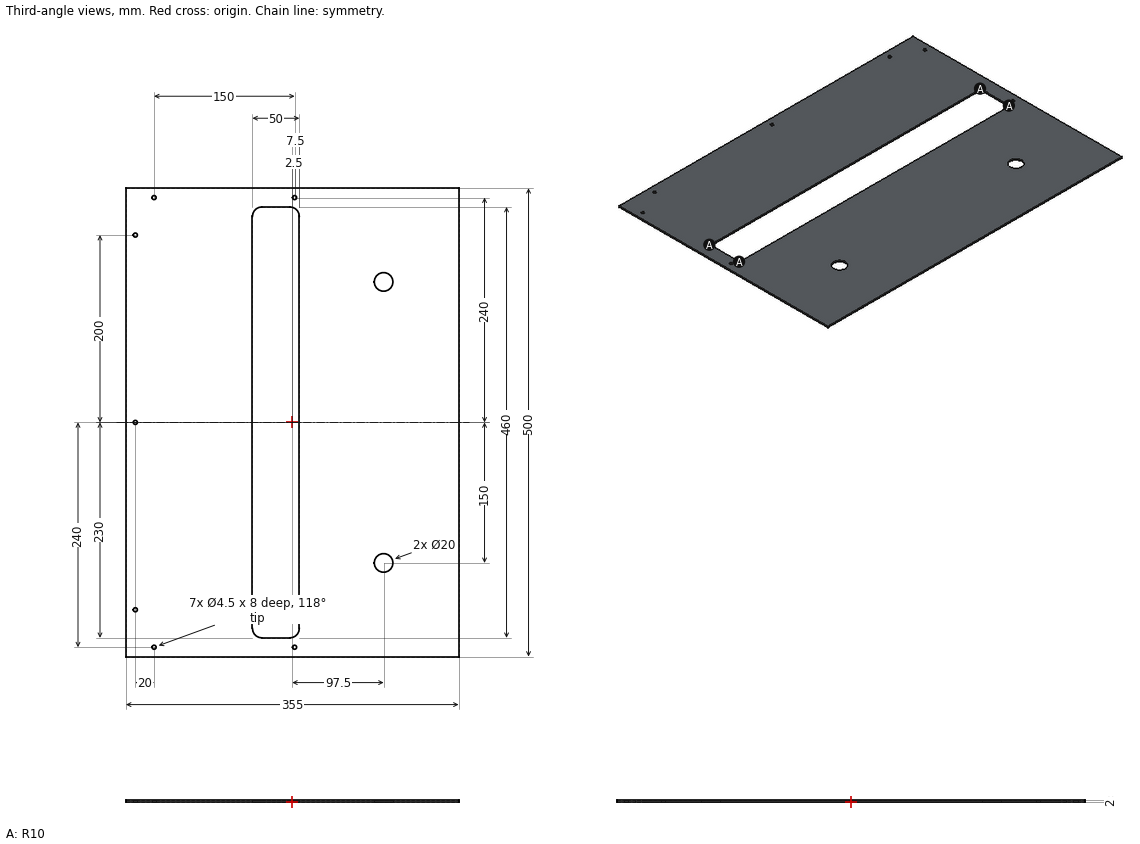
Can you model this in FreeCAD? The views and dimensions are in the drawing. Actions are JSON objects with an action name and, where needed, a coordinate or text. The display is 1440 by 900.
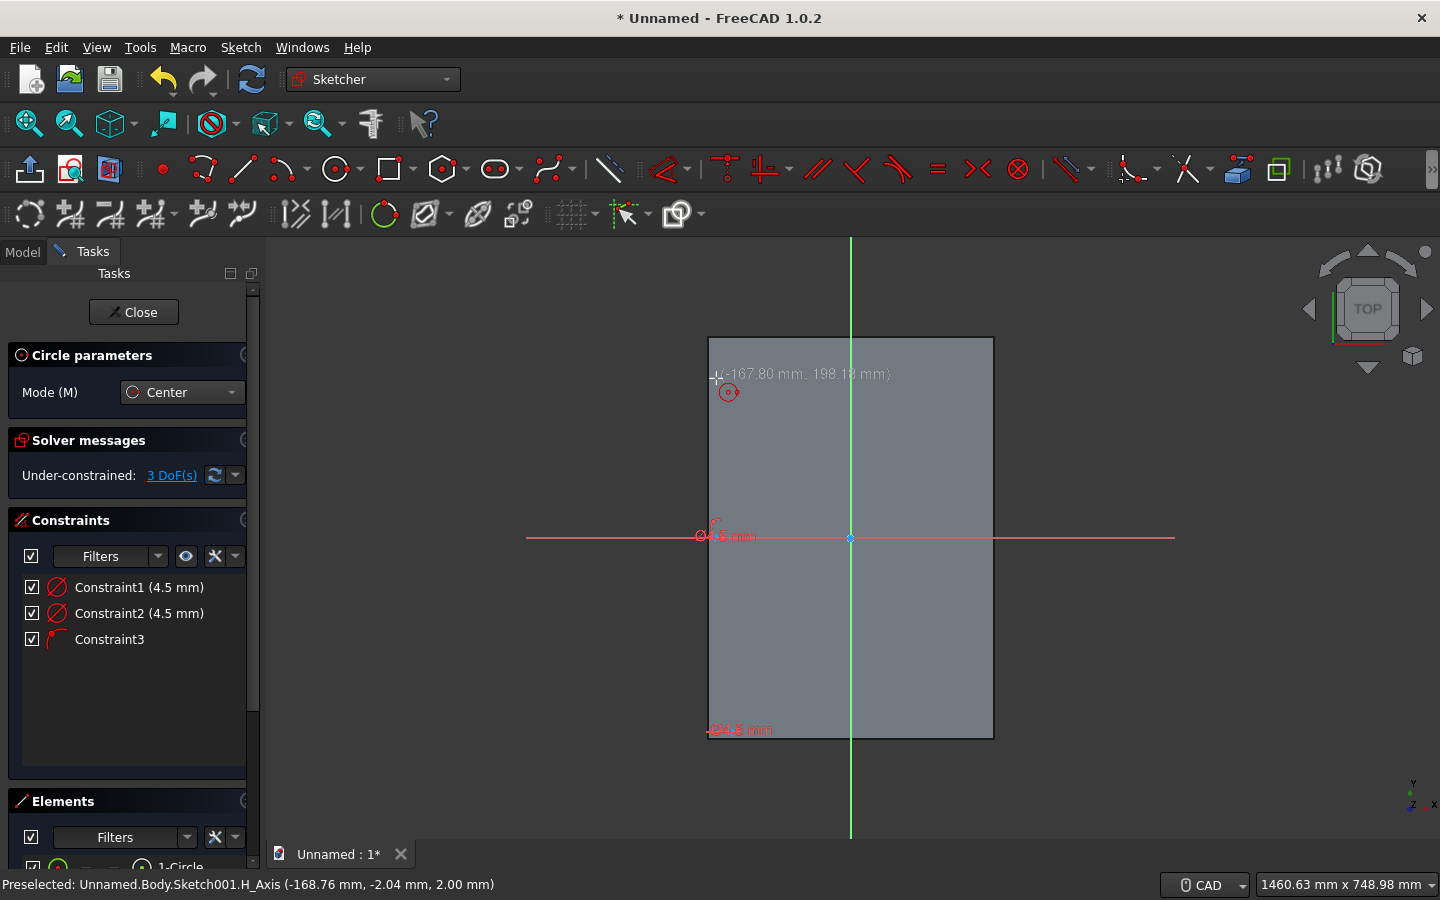
{"action": "left_click", "coordinate": [716, 378]}
{"action": "mouse_move", "coordinate": [718, 376]}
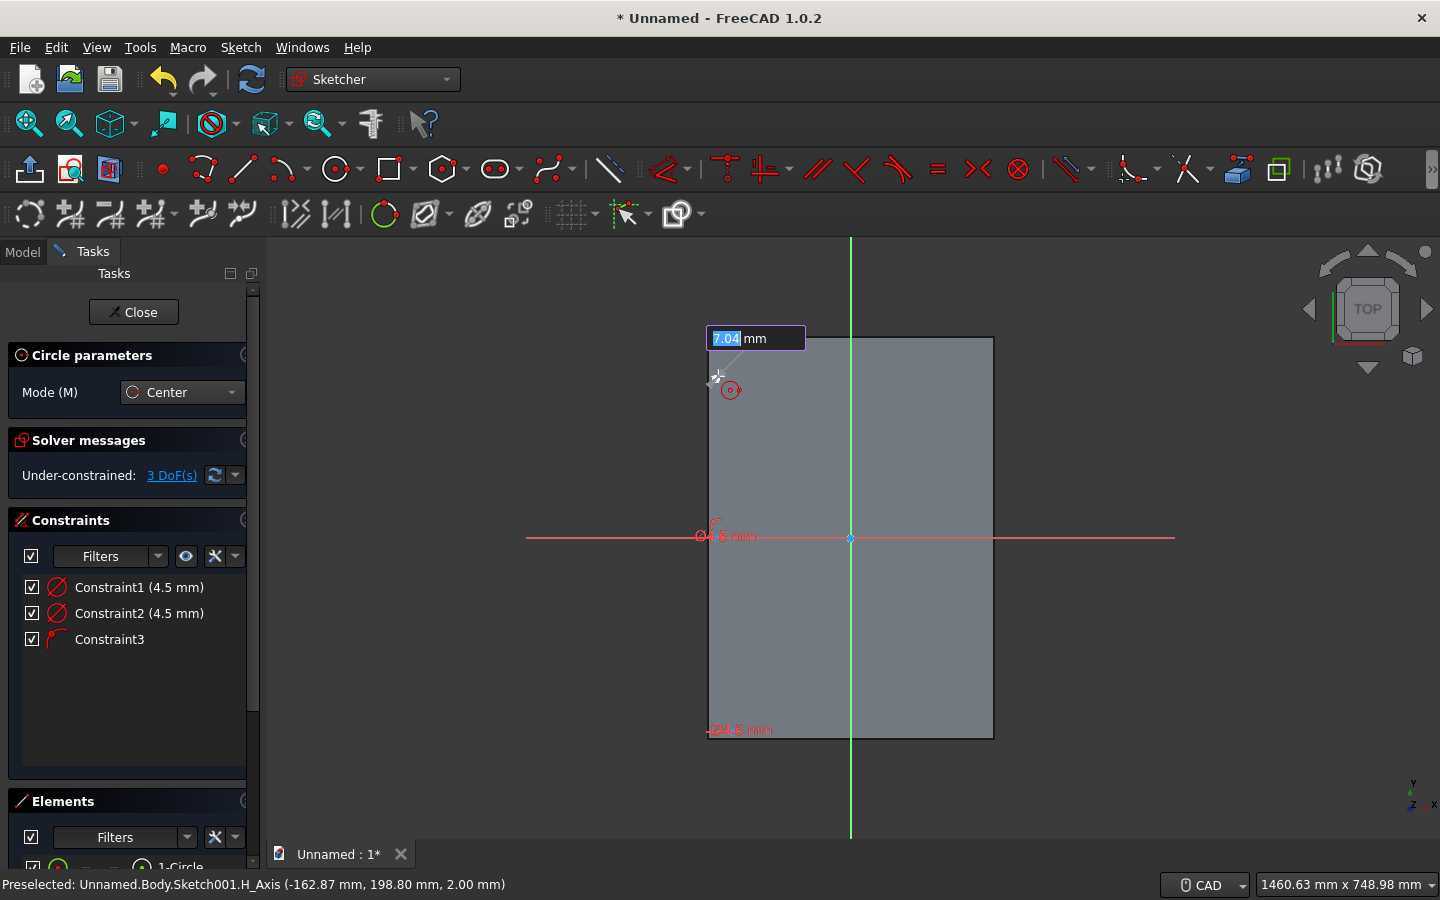
{"action": "type", "text": "4.5"}
{"action": "key", "text": "Return"}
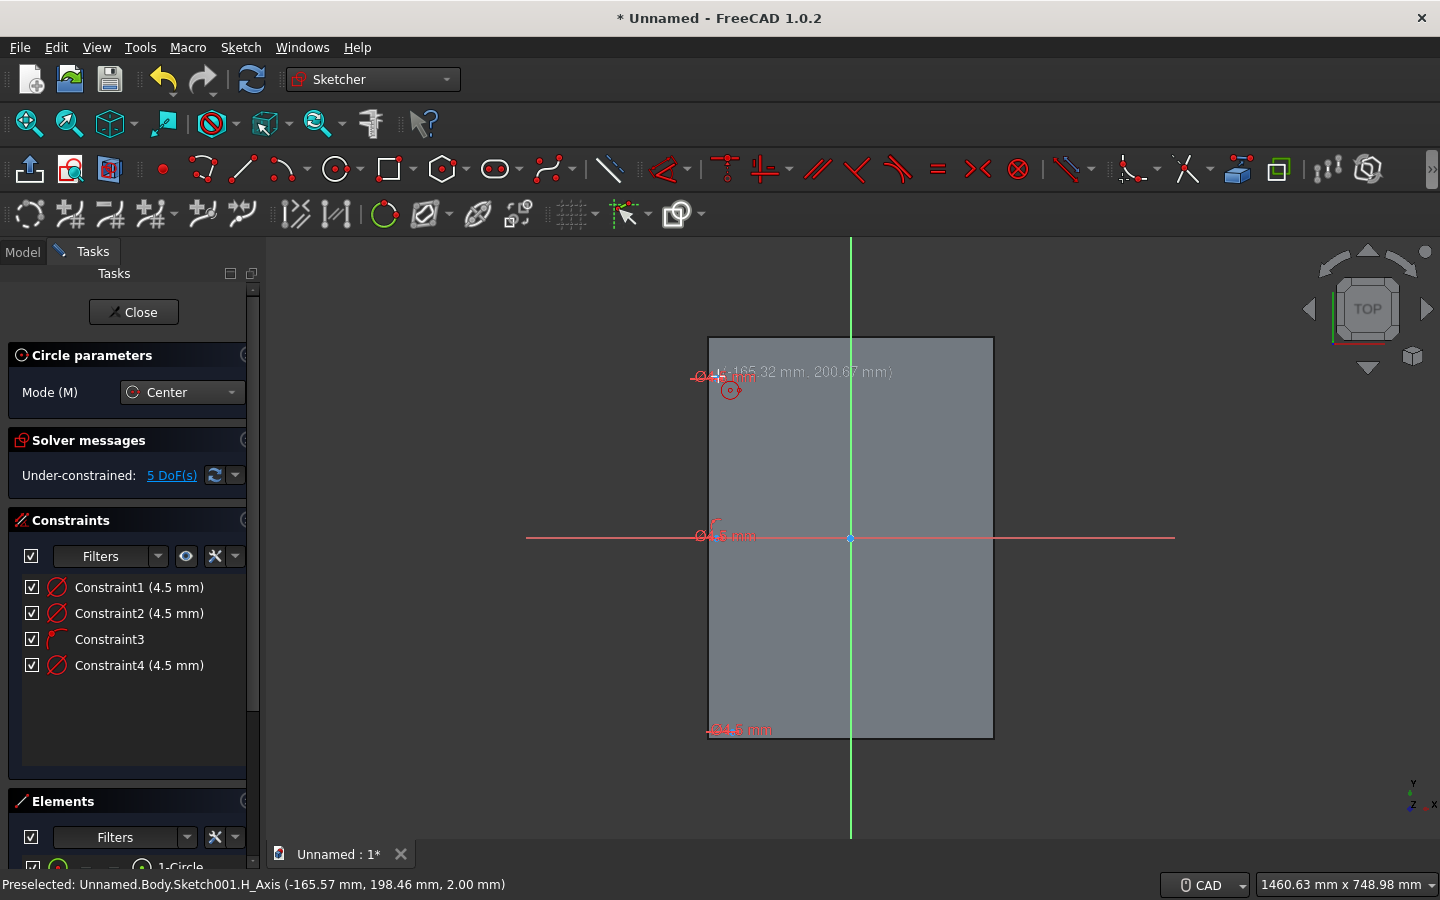
{"action": "scroll", "coordinate": [716, 699], "scroll_direction": "up", "scroll_amount": 13}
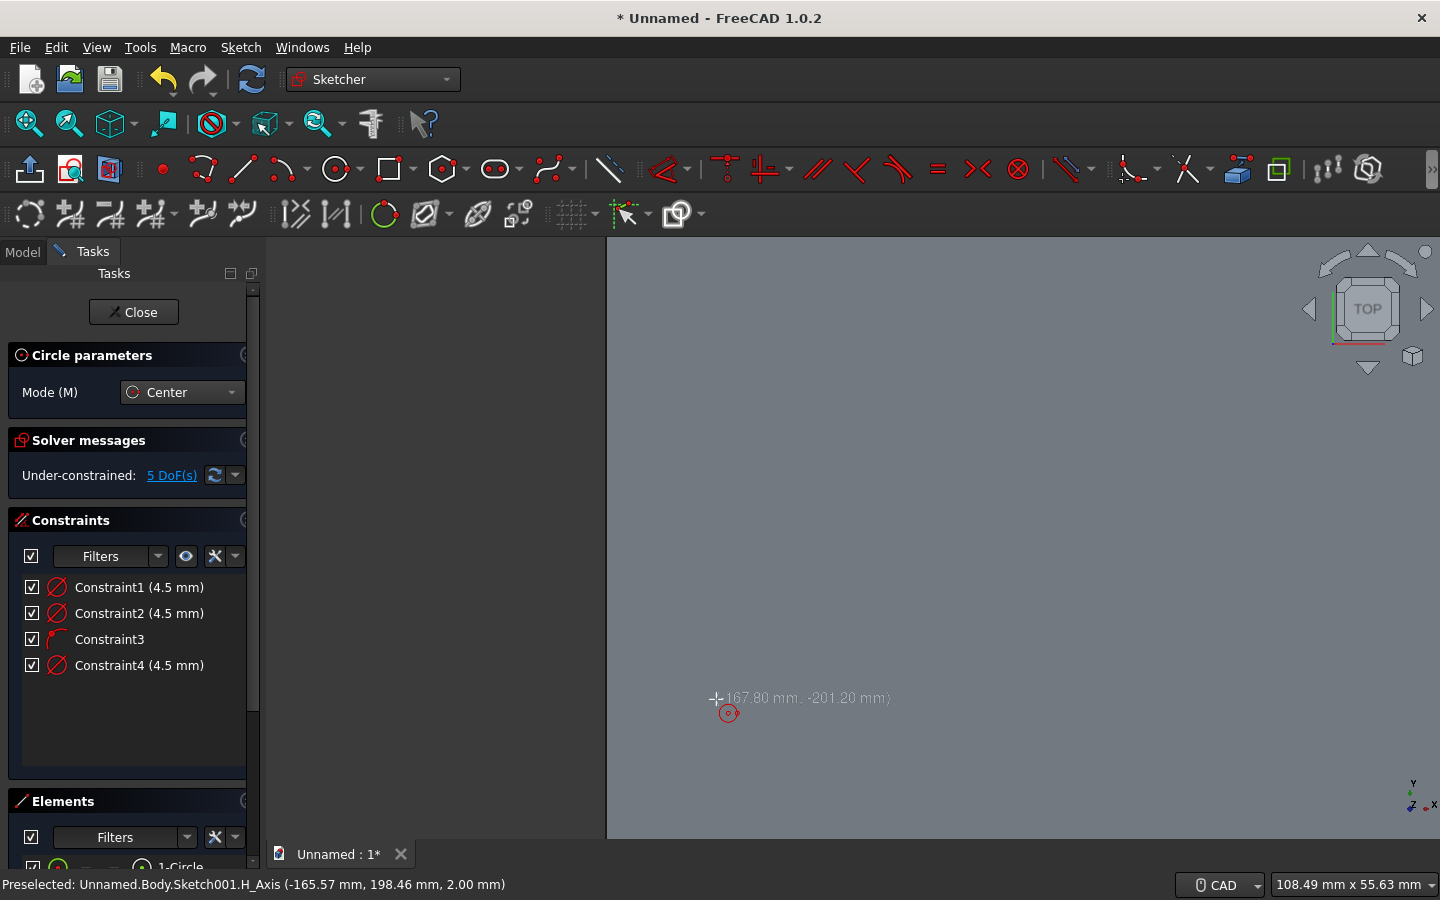
{"action": "scroll", "coordinate": [716, 699], "scroll_direction": "down", "scroll_amount": 13}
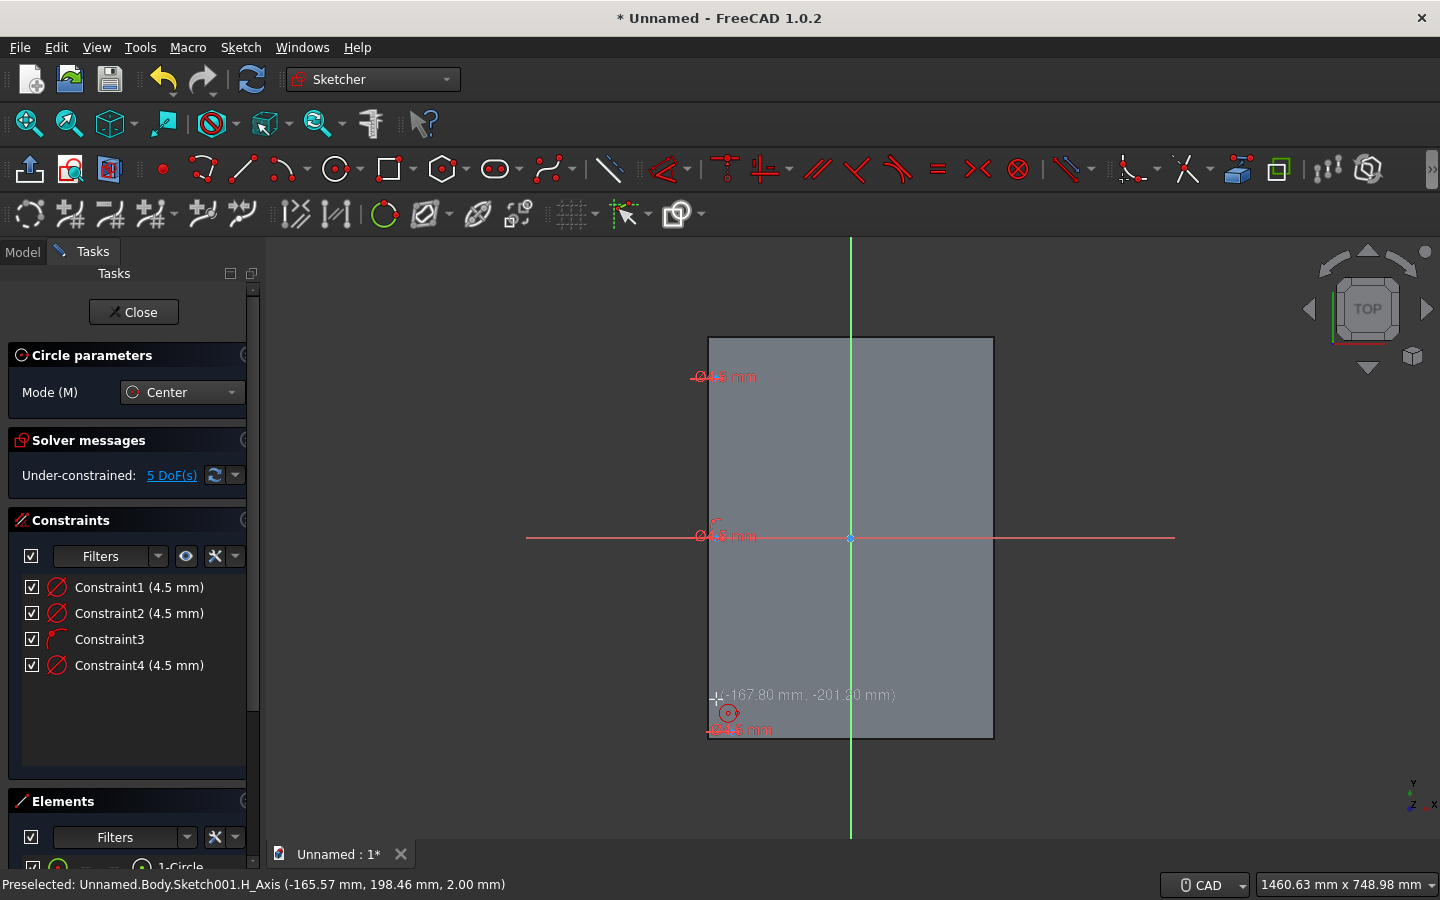
{"action": "left_click", "coordinate": [716, 699]}
{"action": "mouse_move", "coordinate": [718, 698]}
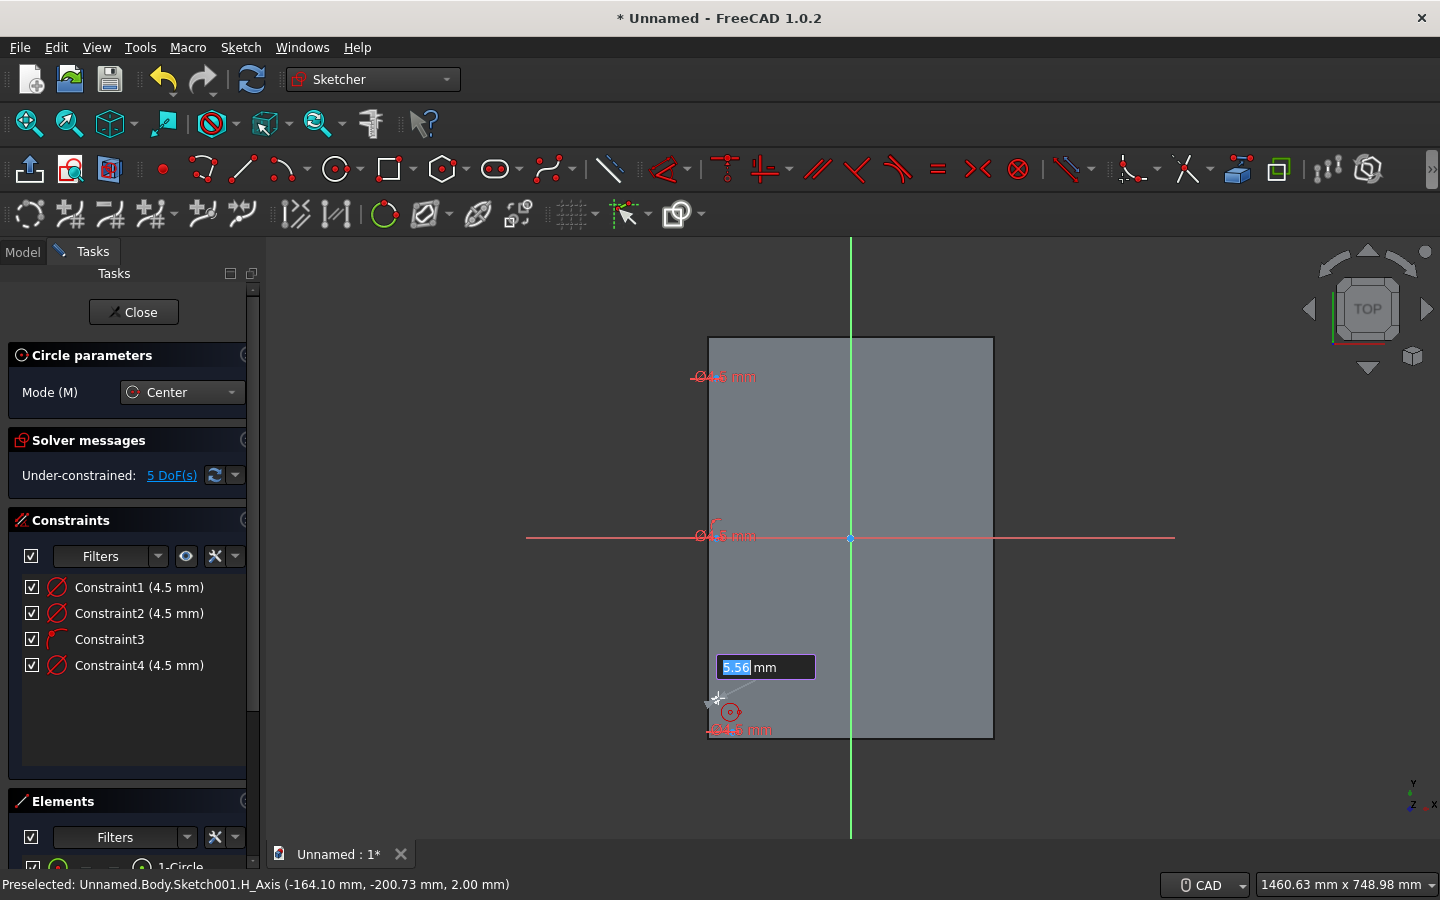
{"action": "type", "text": "4.5"}
{"action": "key", "text": "Return"}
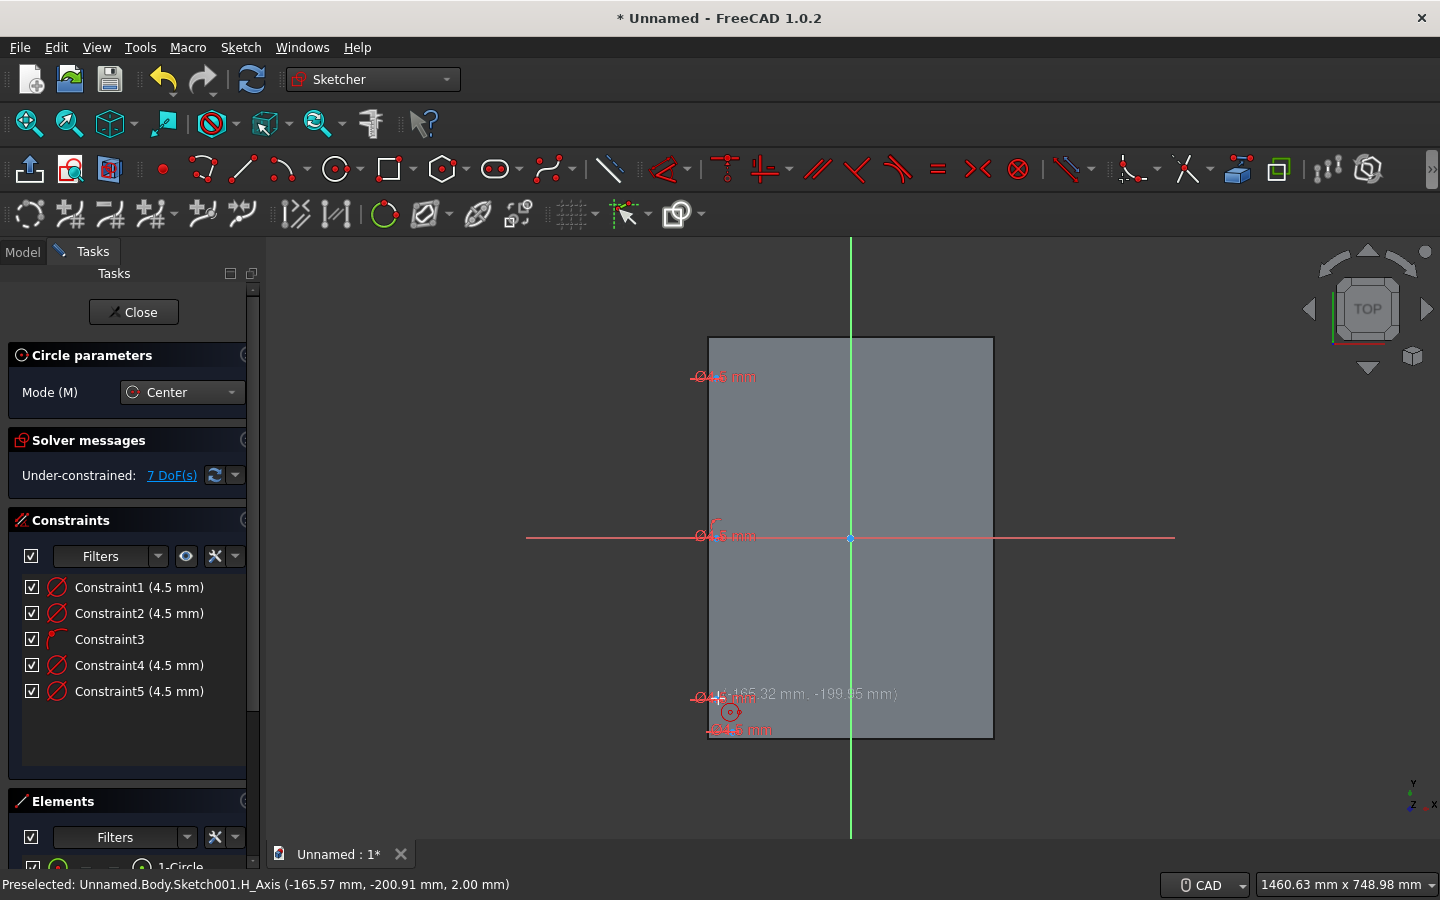
{"action": "scroll", "coordinate": [732, 345], "scroll_direction": "up", "scroll_amount": 13}